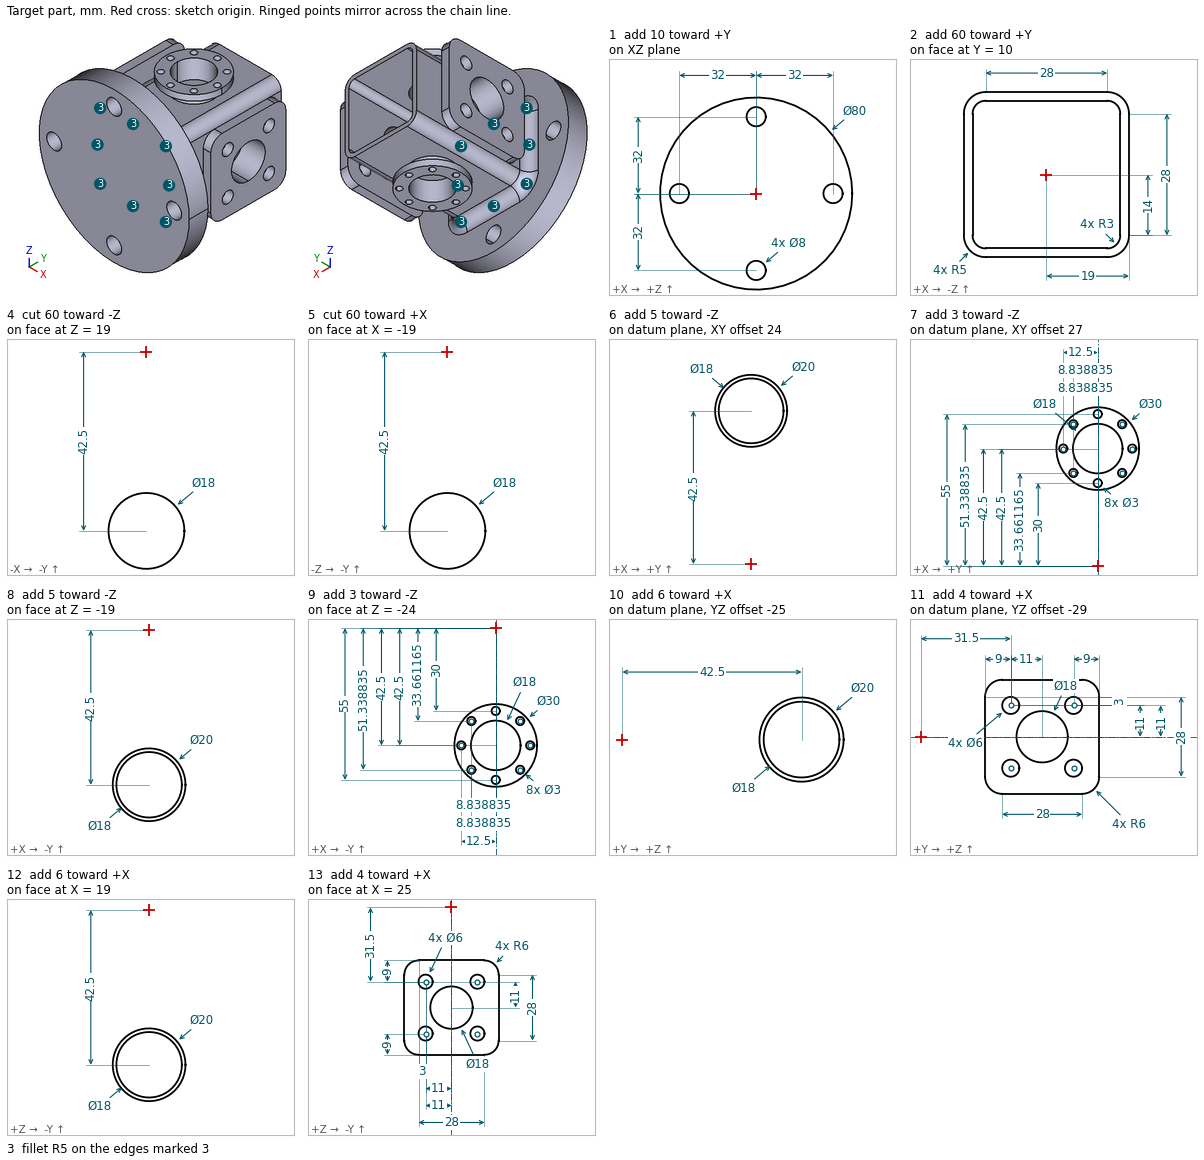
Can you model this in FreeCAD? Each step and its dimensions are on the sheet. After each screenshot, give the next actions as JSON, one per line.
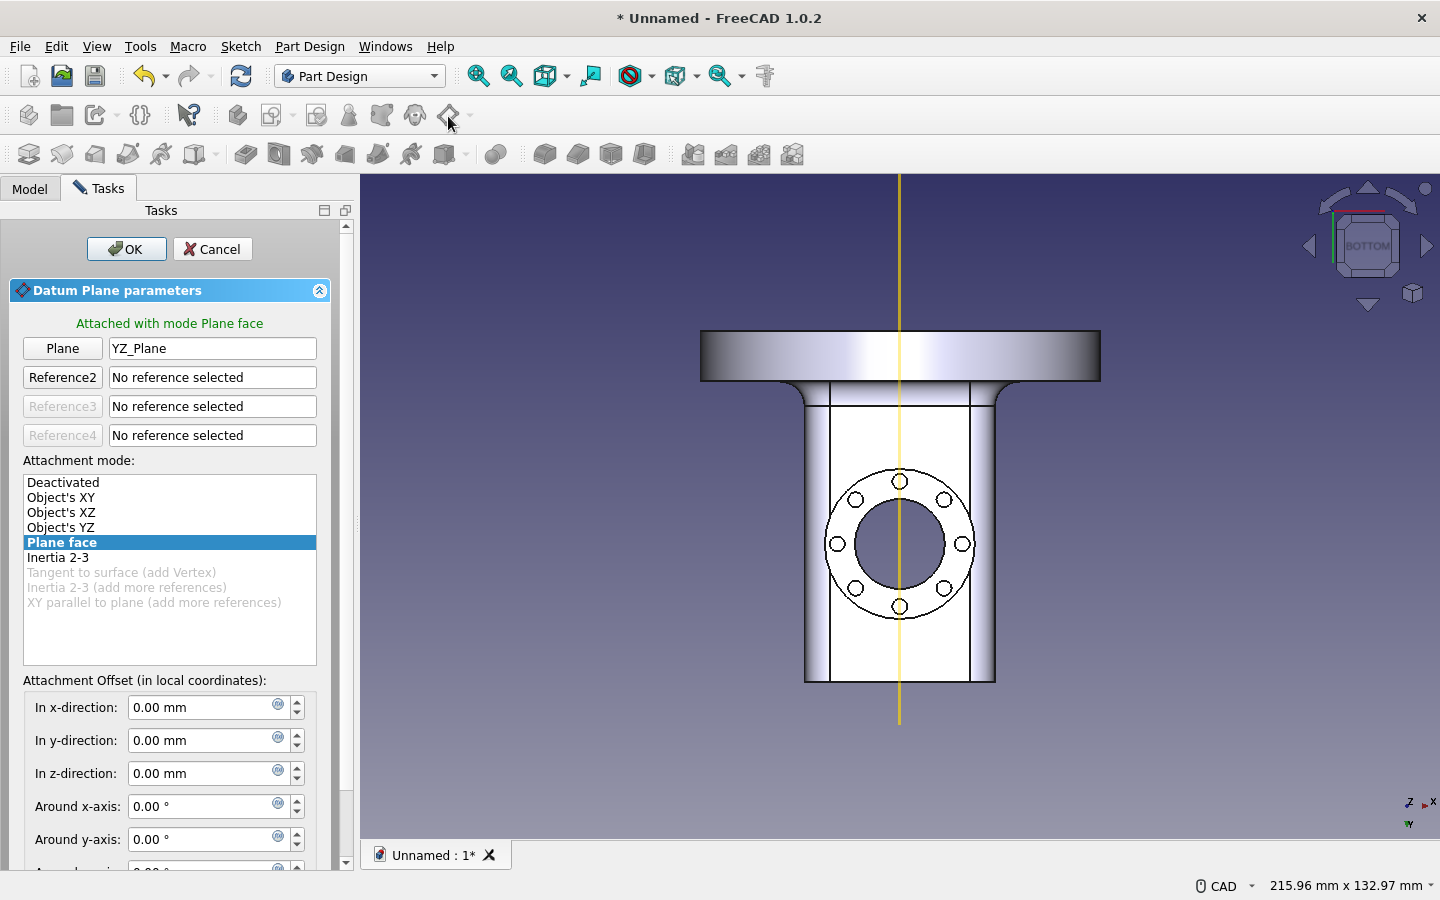
{"action": "triple_click", "coordinate": [210, 774]}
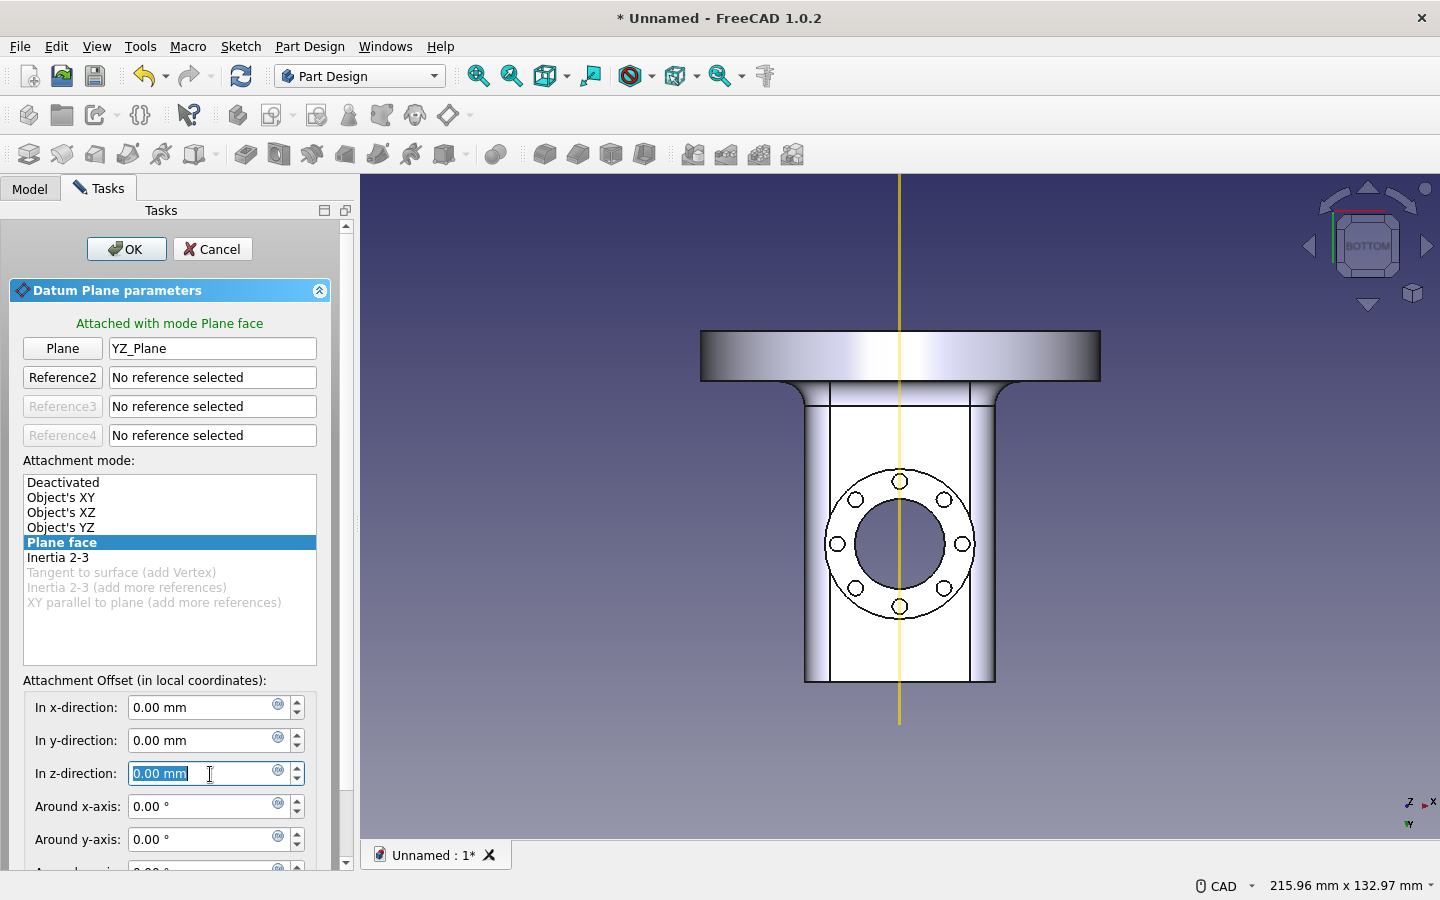
{"action": "type", "text": "-25"}
{"action": "key", "text": "Tab"}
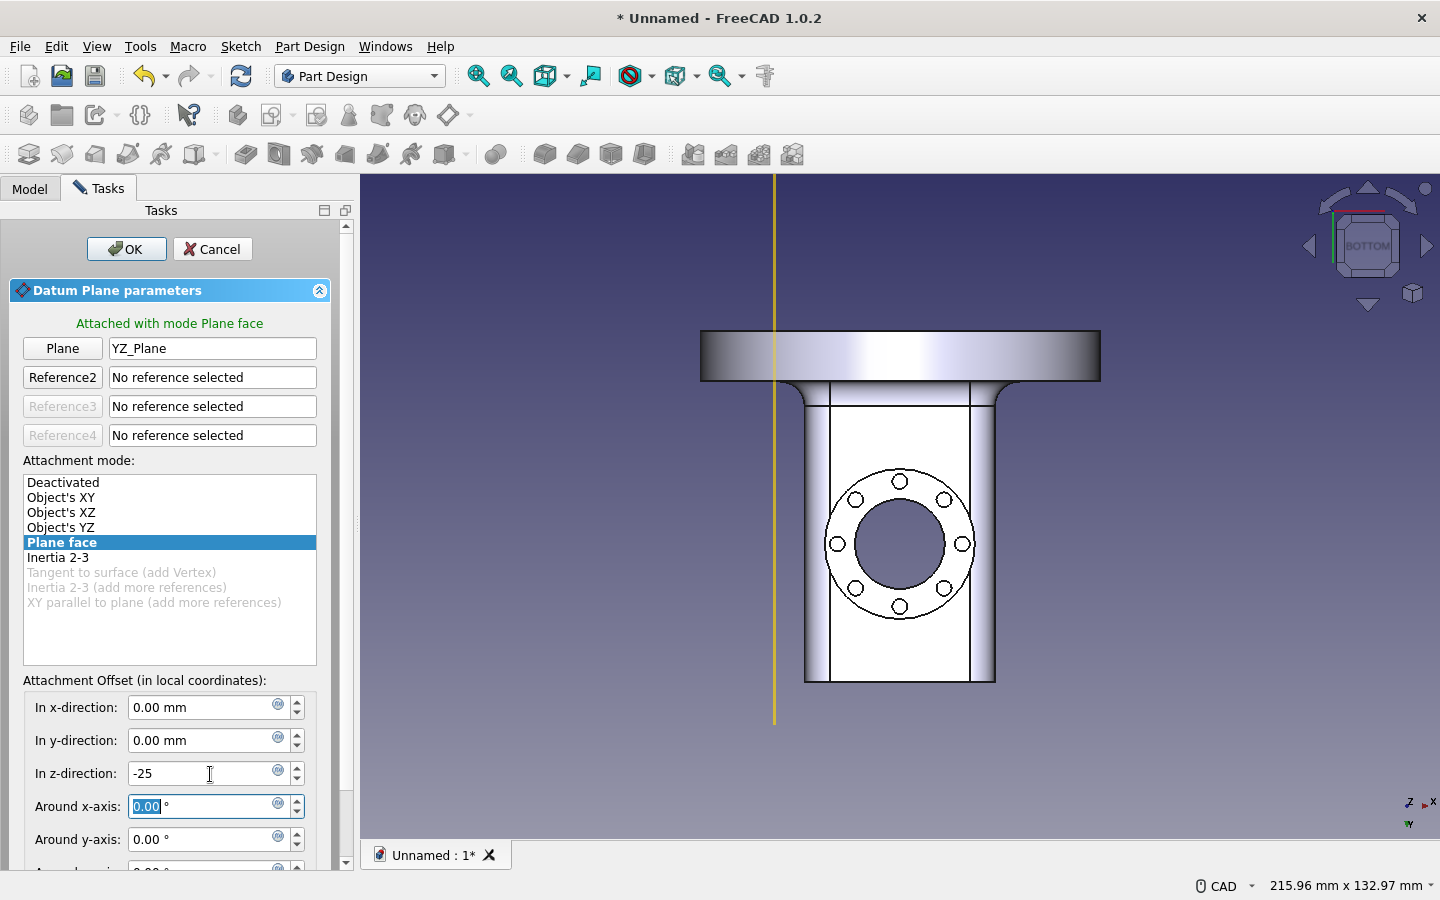
{"action": "left_click", "coordinate": [127, 249]}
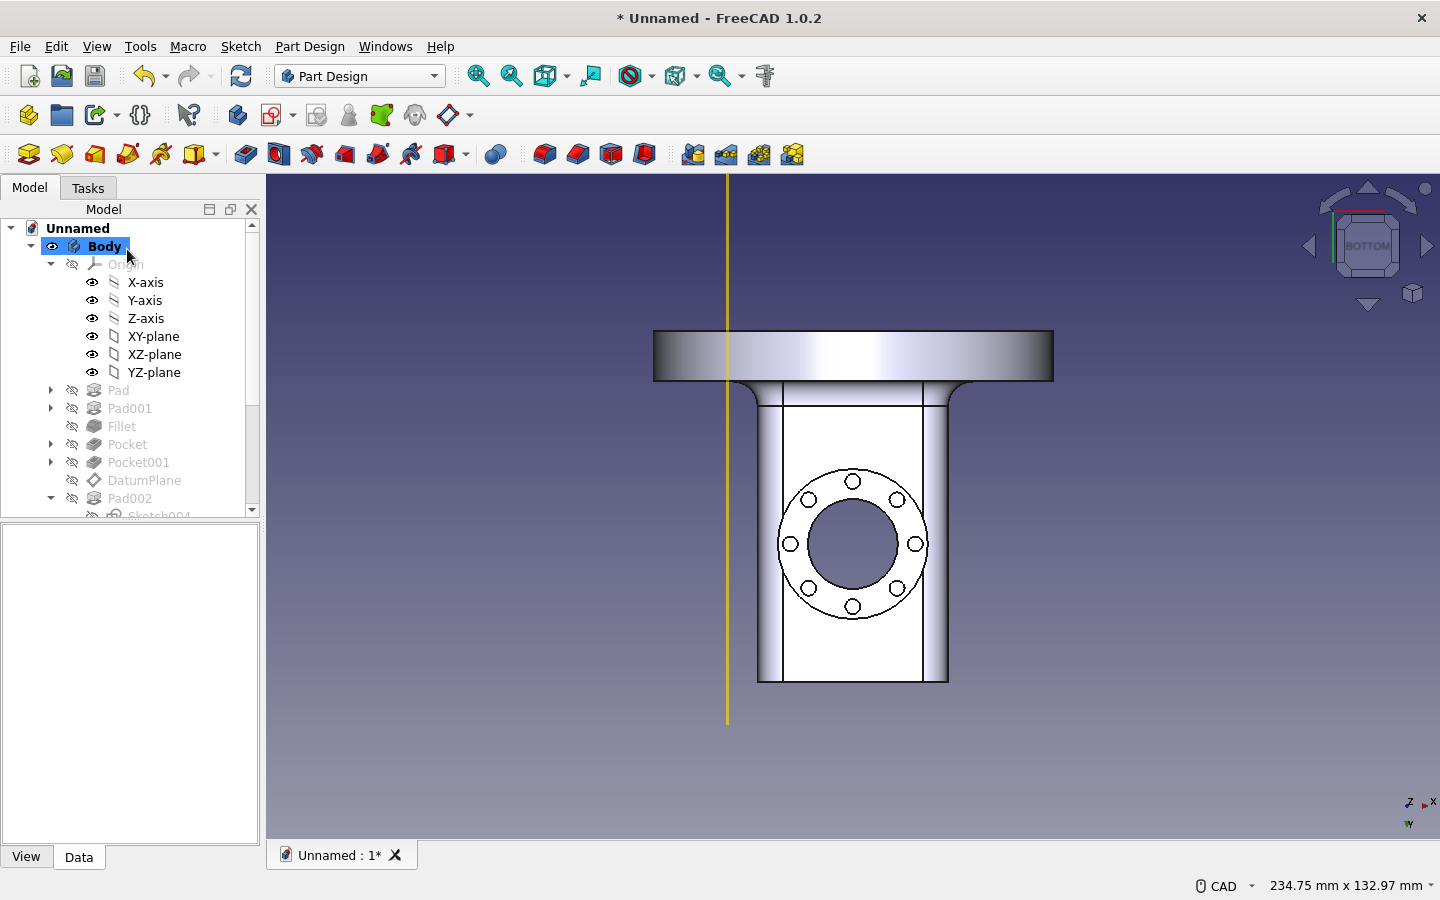
{"action": "scroll", "coordinate": [101, 368], "scroll_direction": "down", "scroll_amount": 3}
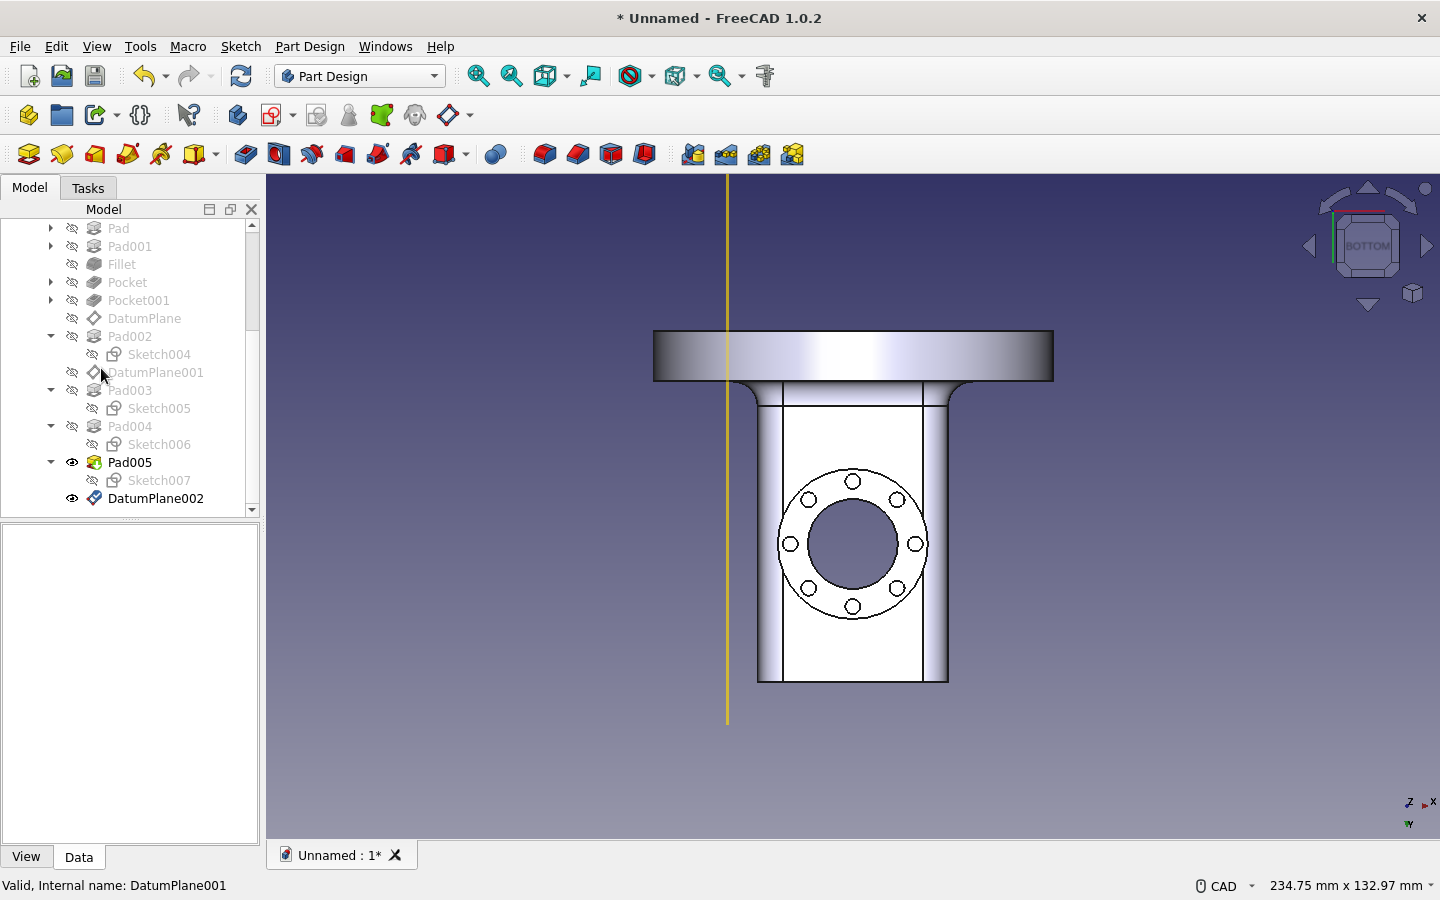
{"action": "left_click", "coordinate": [117, 498]}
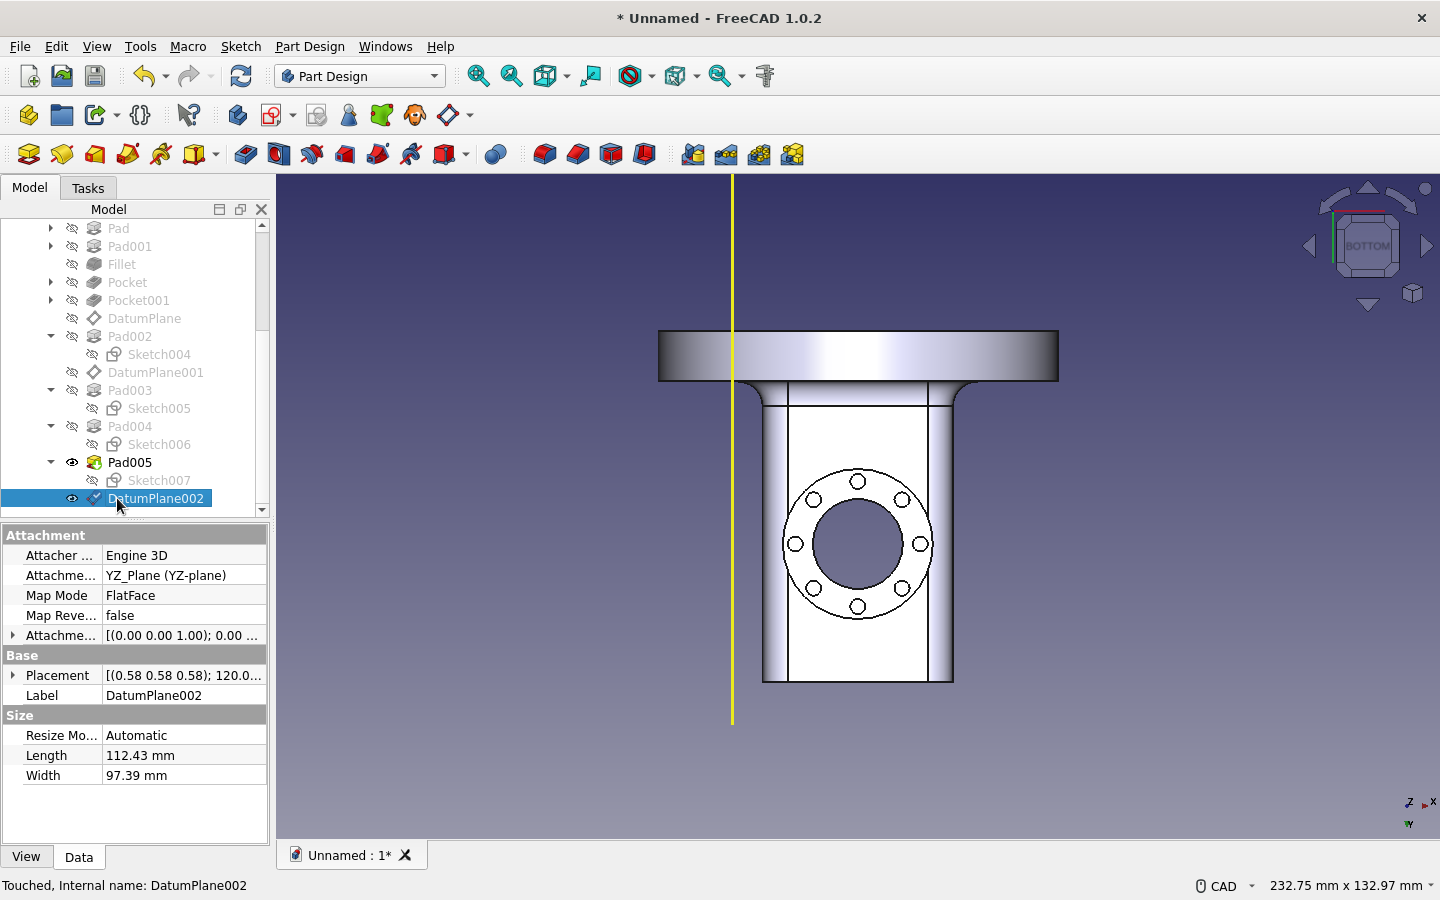
{"action": "left_click", "coordinate": [270, 116]}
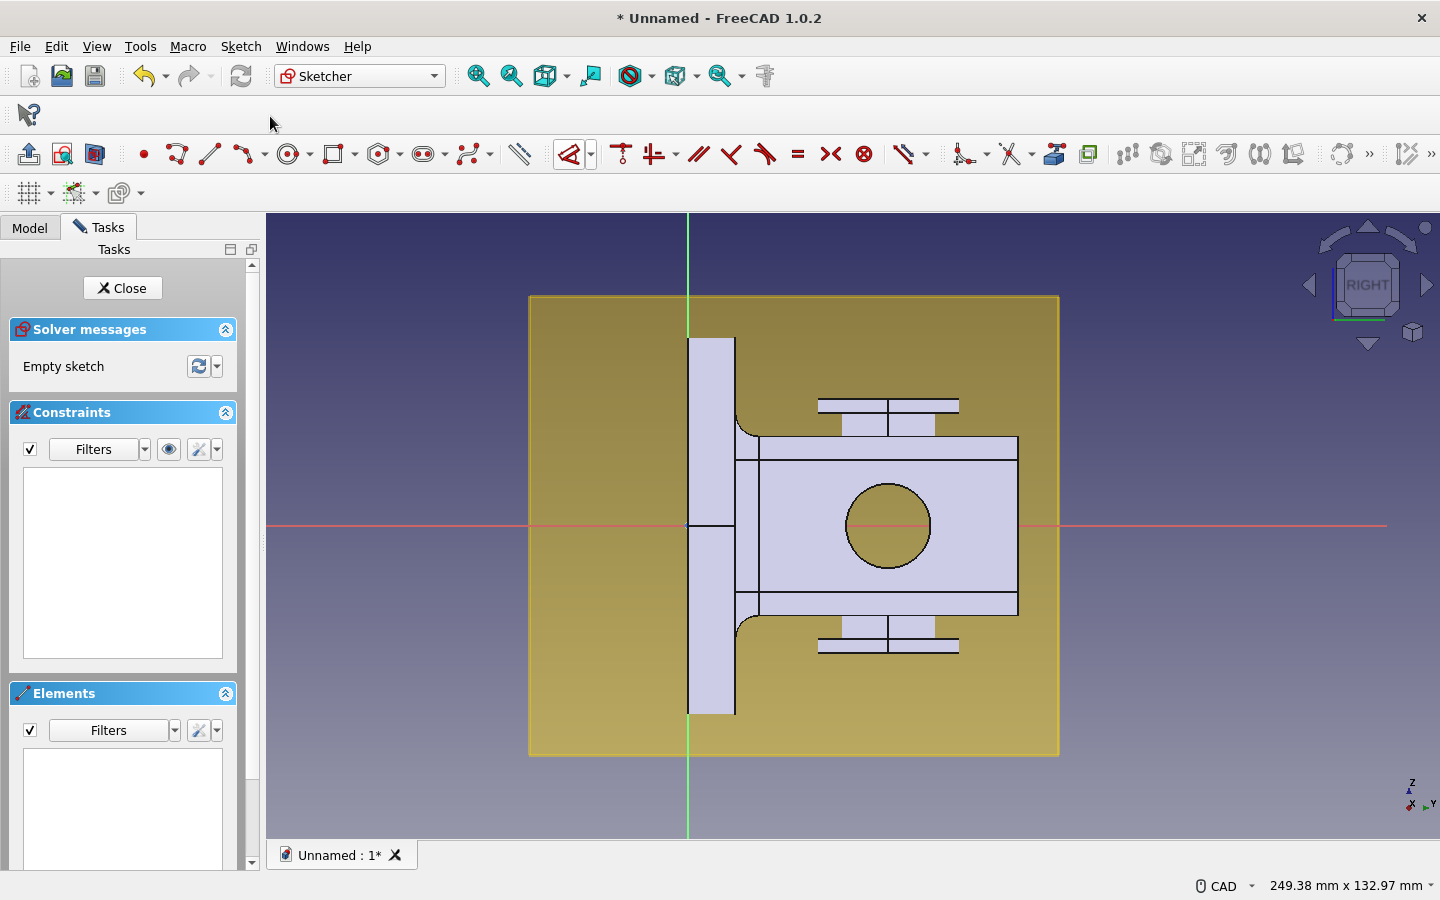
{"action": "key", "text": "q s"}